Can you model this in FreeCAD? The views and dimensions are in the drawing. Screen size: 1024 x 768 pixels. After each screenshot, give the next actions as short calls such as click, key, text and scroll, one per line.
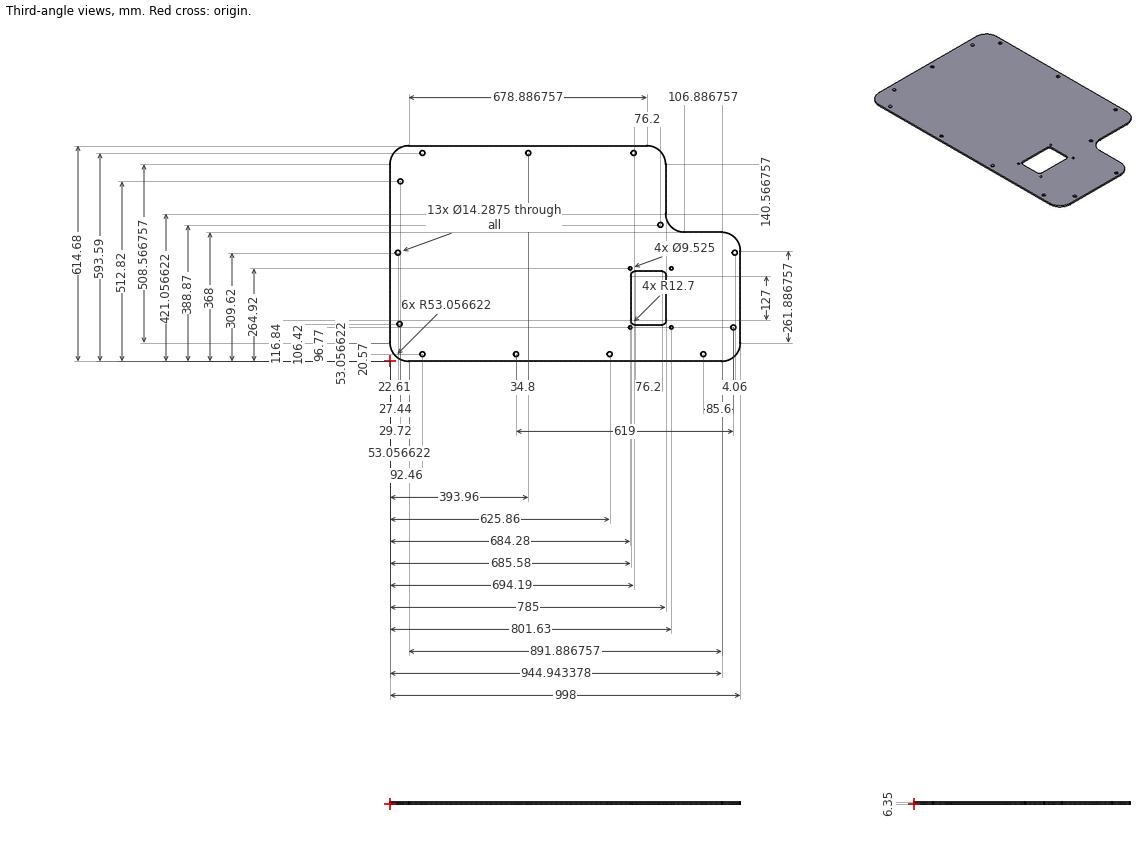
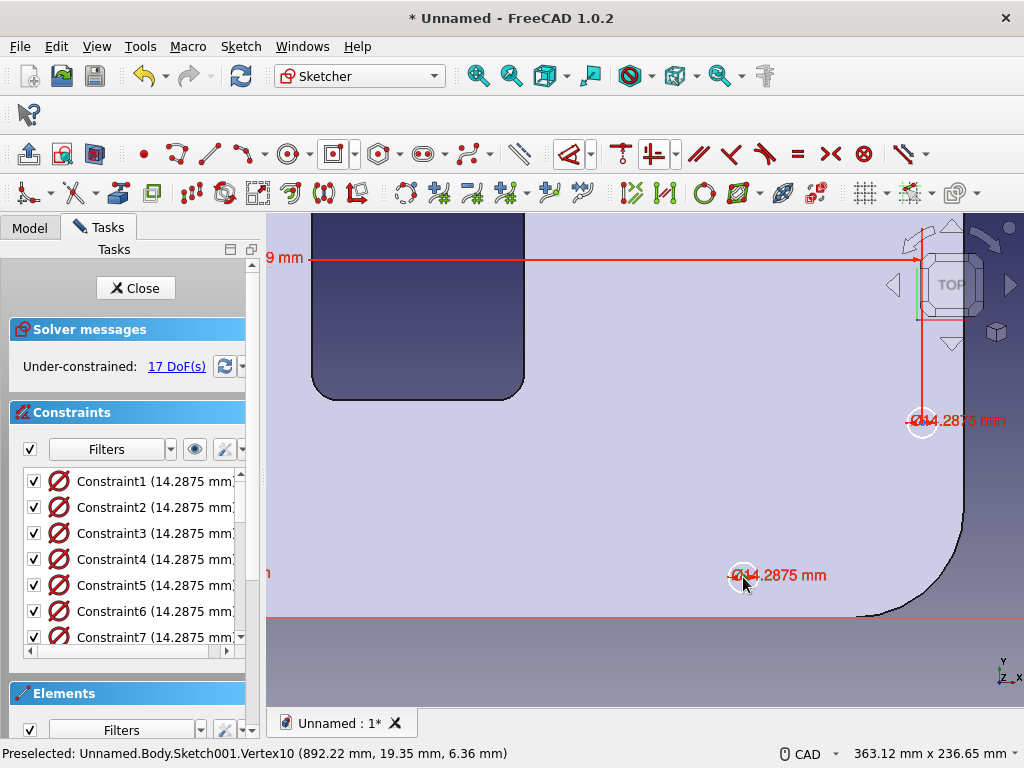
click(590, 154)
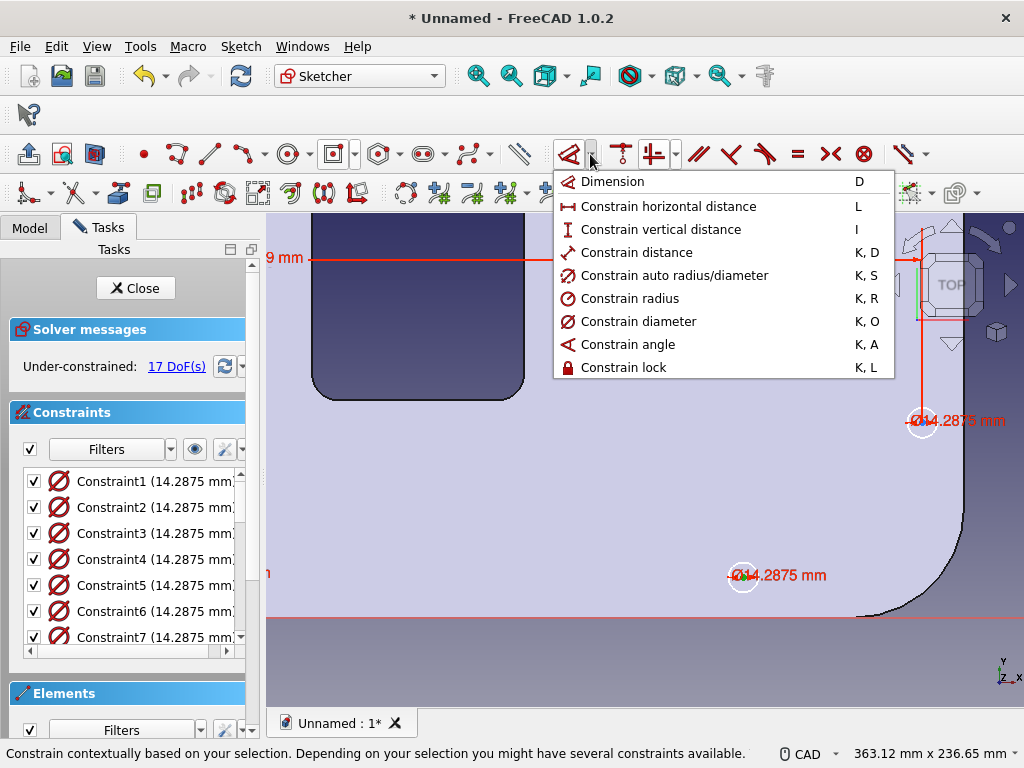
click(724, 230)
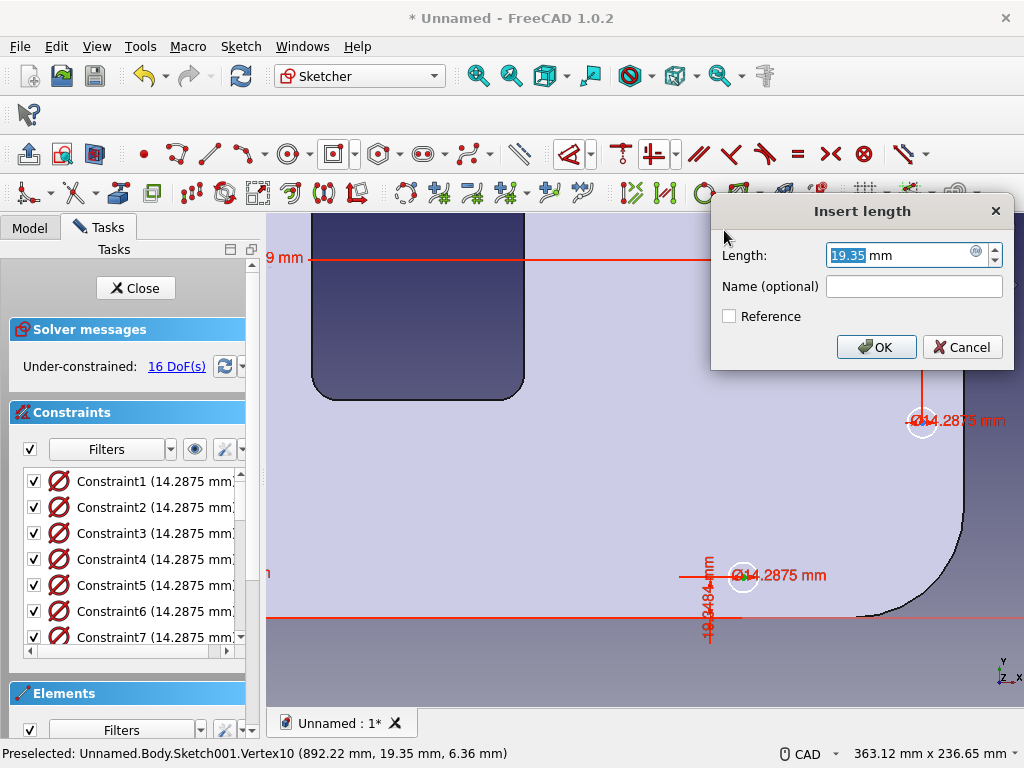
text(20.57)
key(Return)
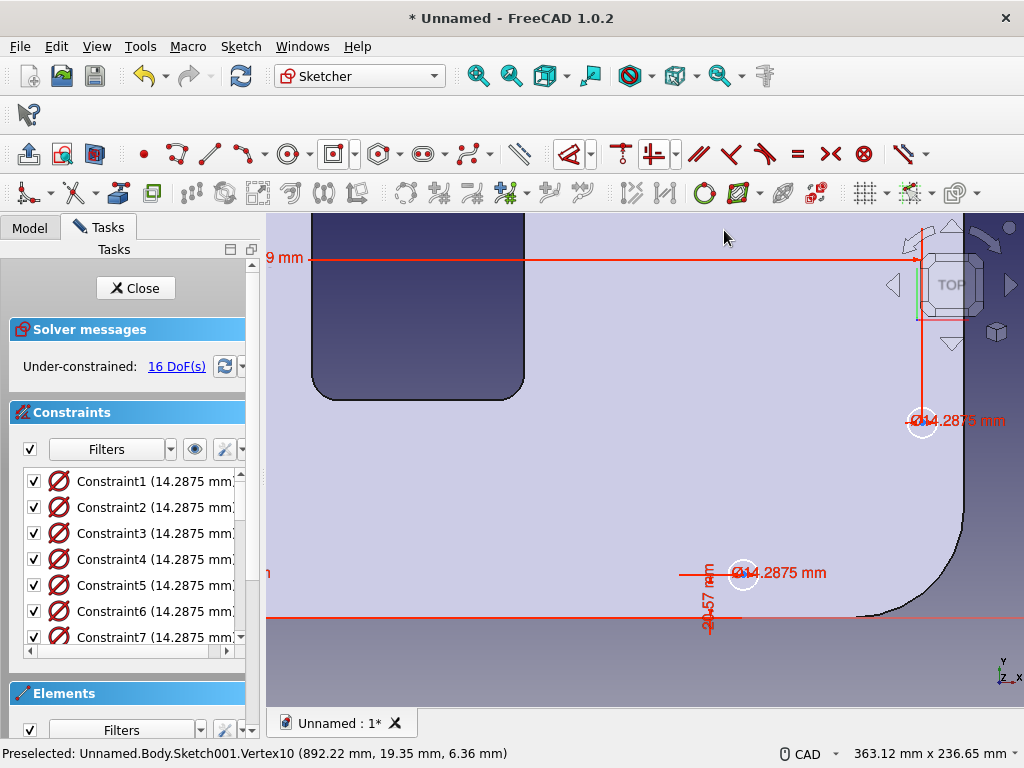
scroll(744, 579, down, 8)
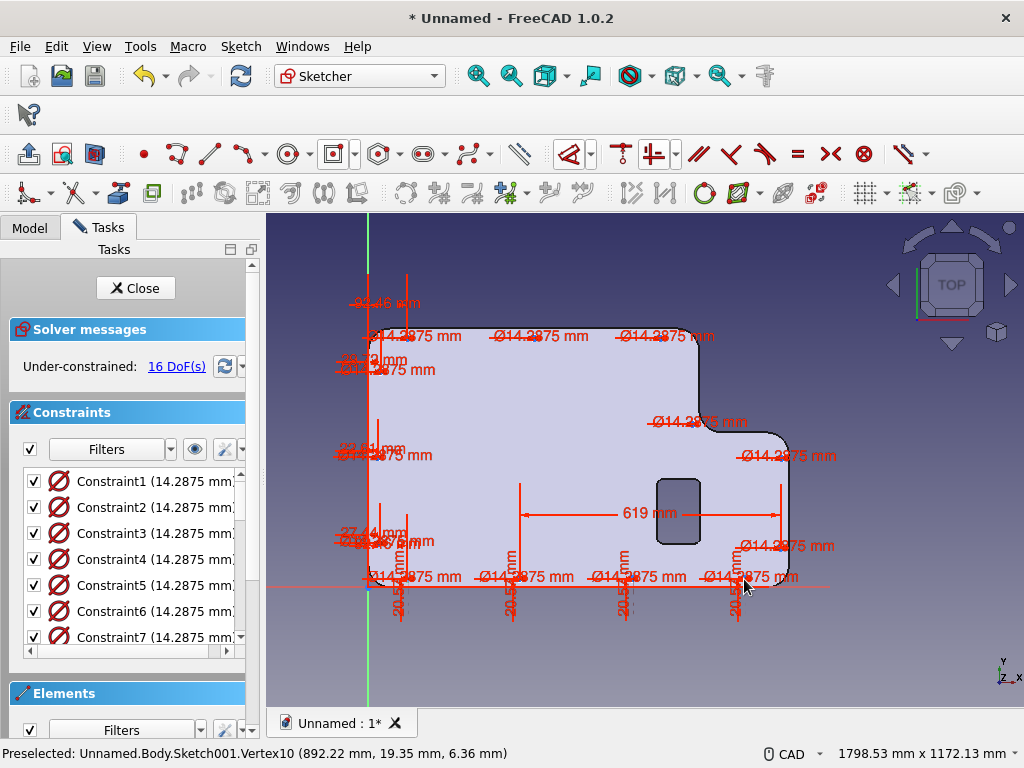
click(781, 548)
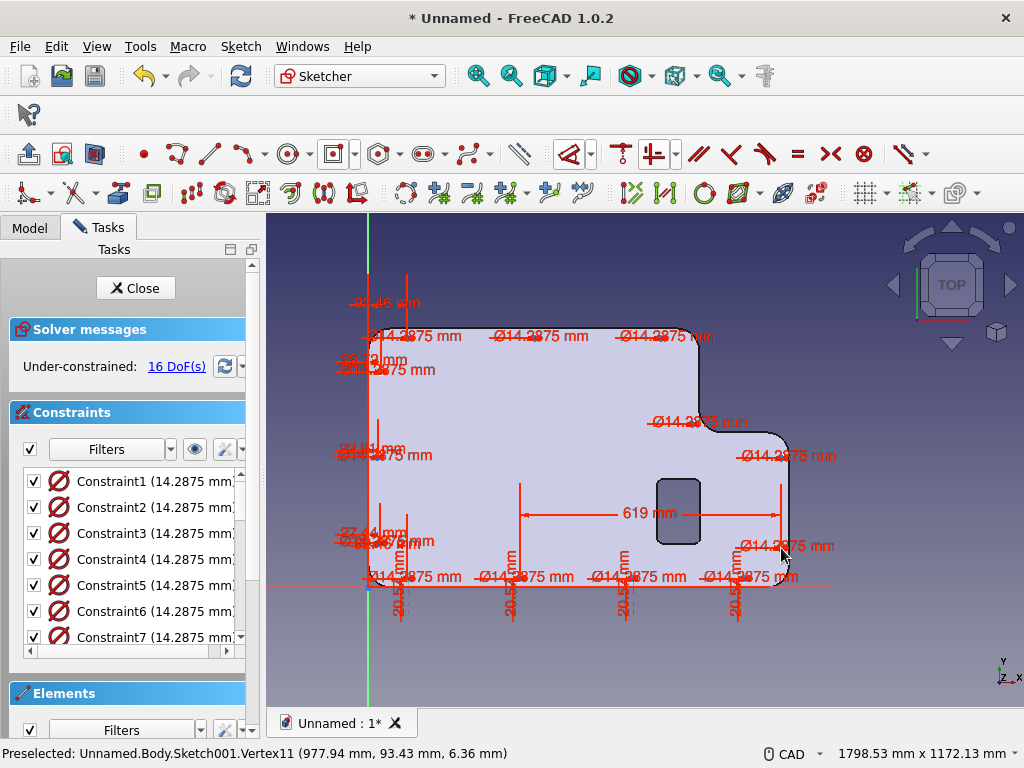
click(590, 154)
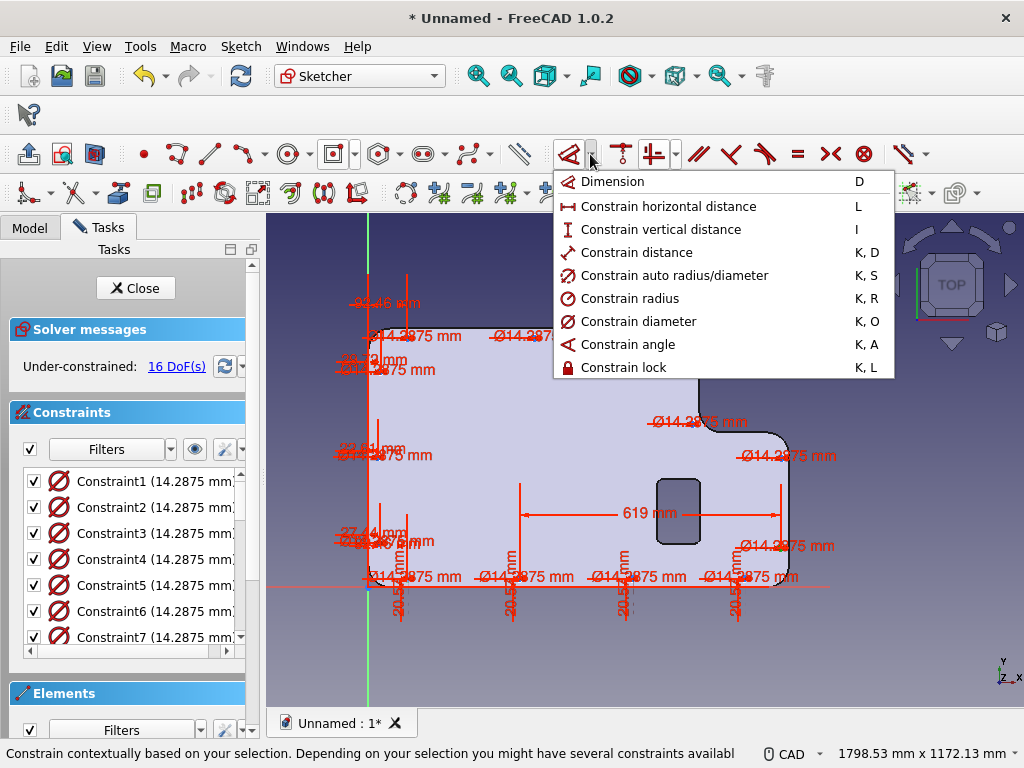
click(724, 230)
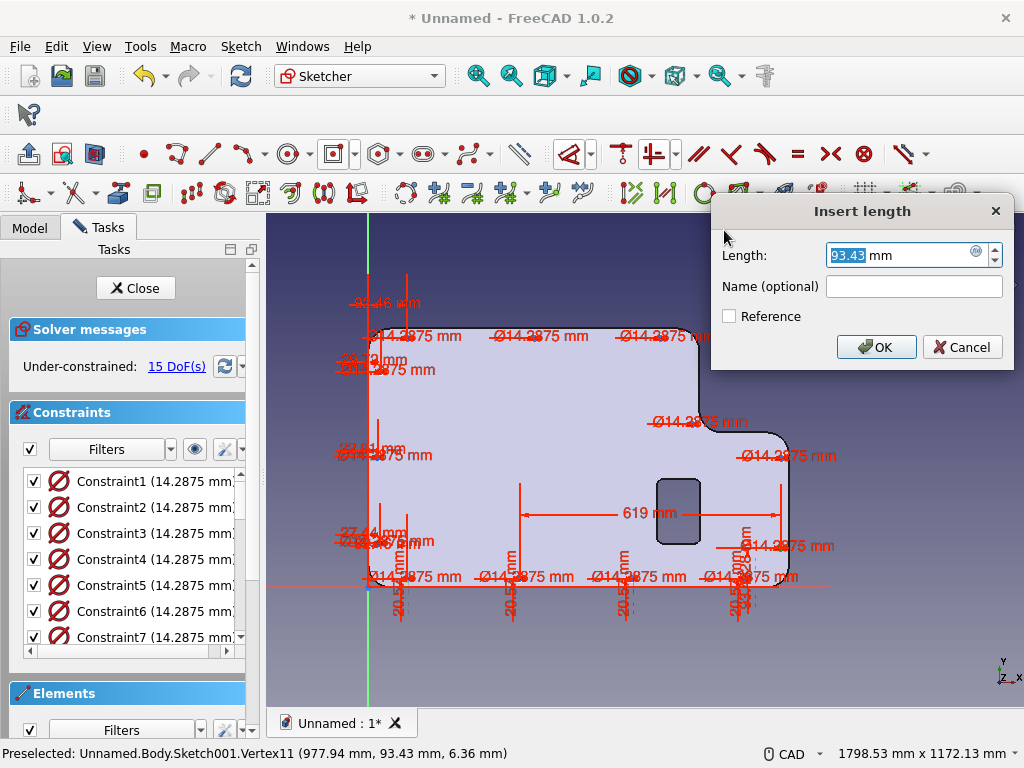
text(96.77)
key(Return)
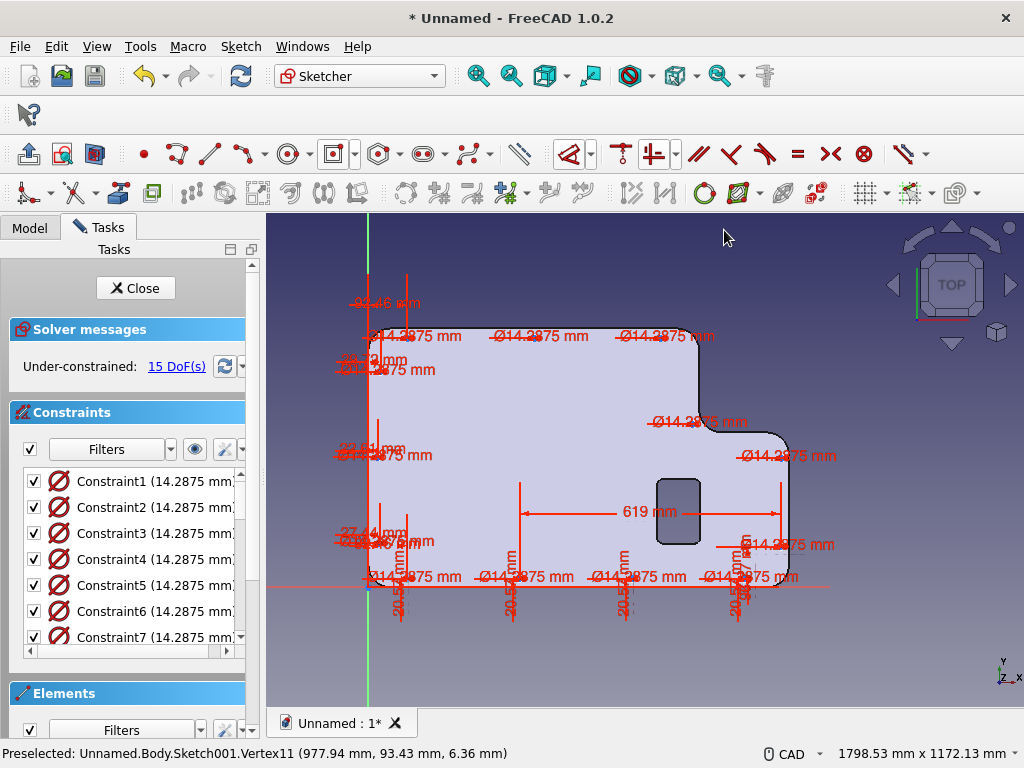
scroll(534, 338, up, 5)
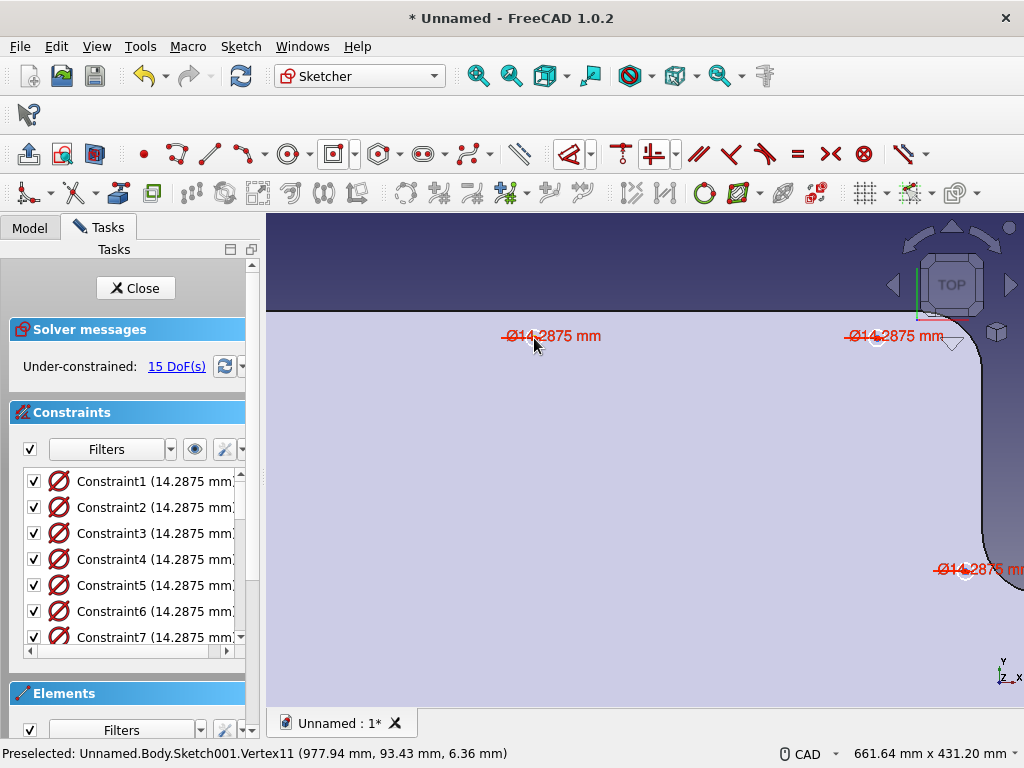
click(534, 338)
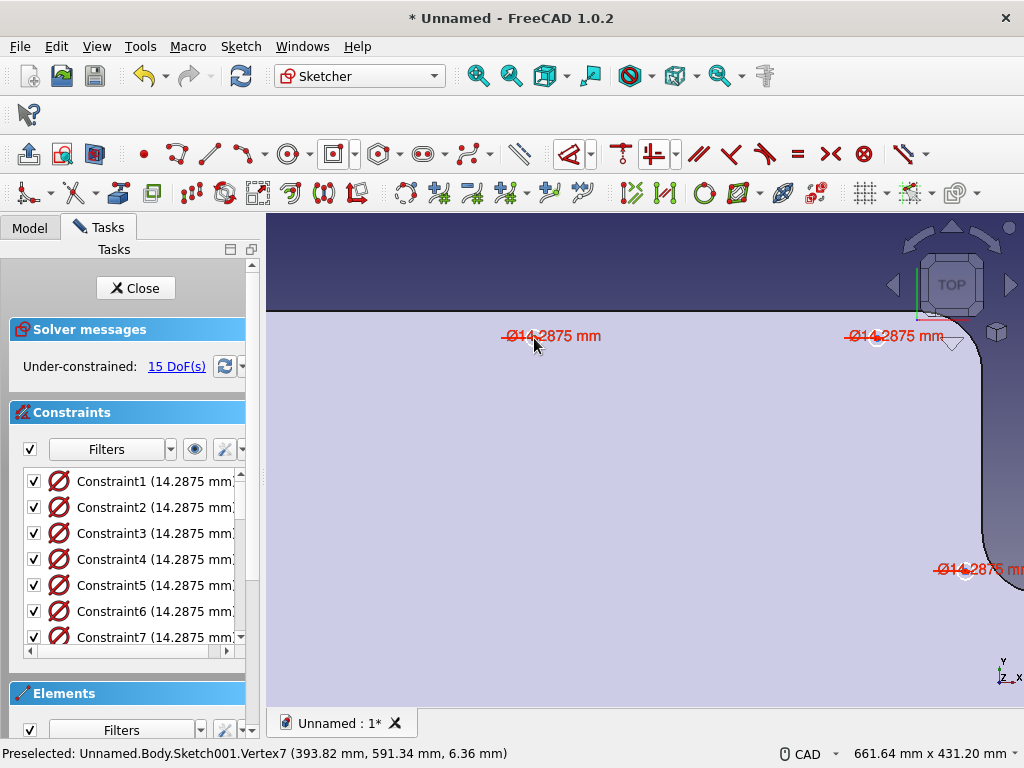
scroll(534, 337, down, 5)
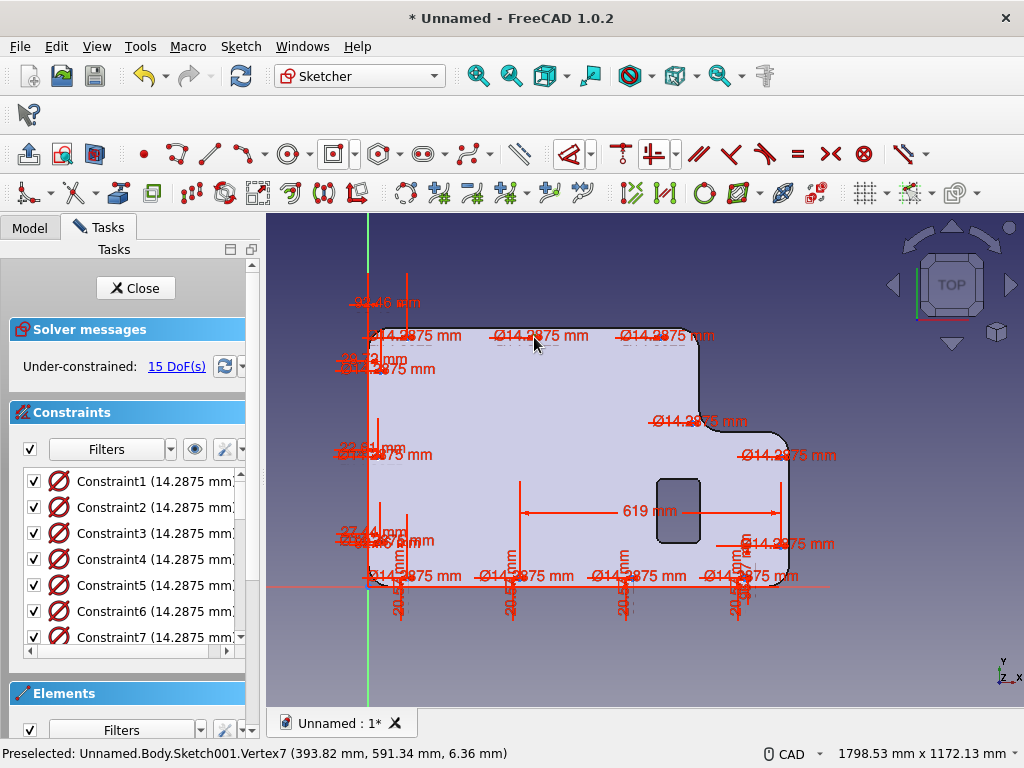
scroll(520, 578, up, 5)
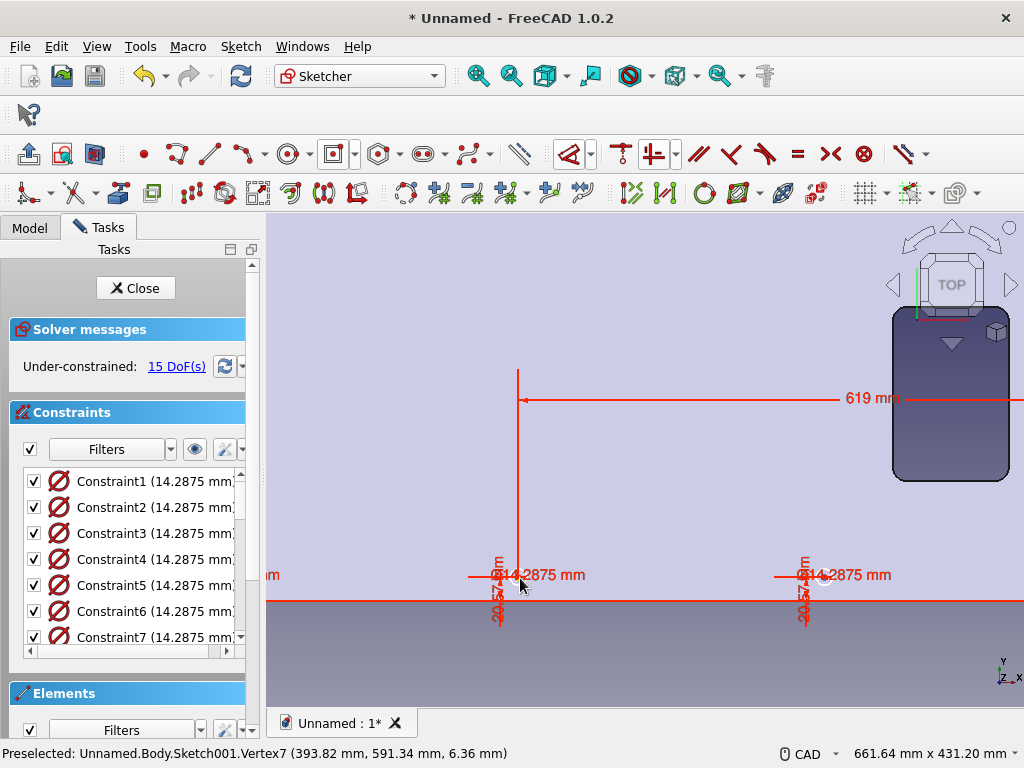
click(518, 577)